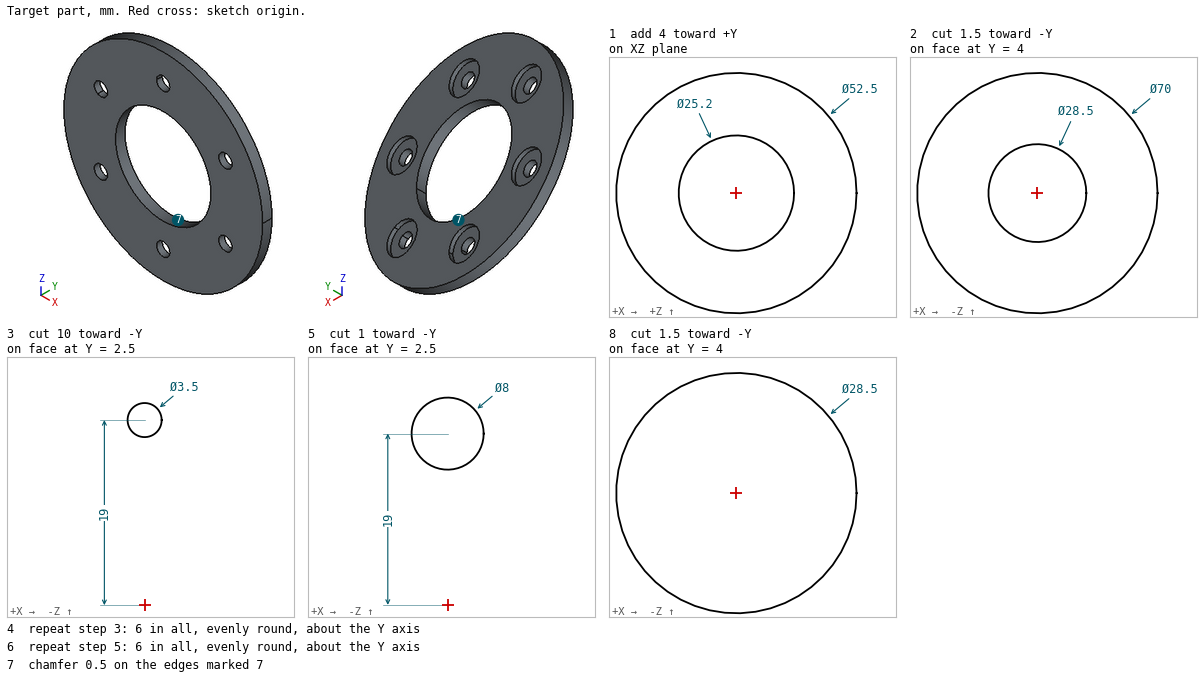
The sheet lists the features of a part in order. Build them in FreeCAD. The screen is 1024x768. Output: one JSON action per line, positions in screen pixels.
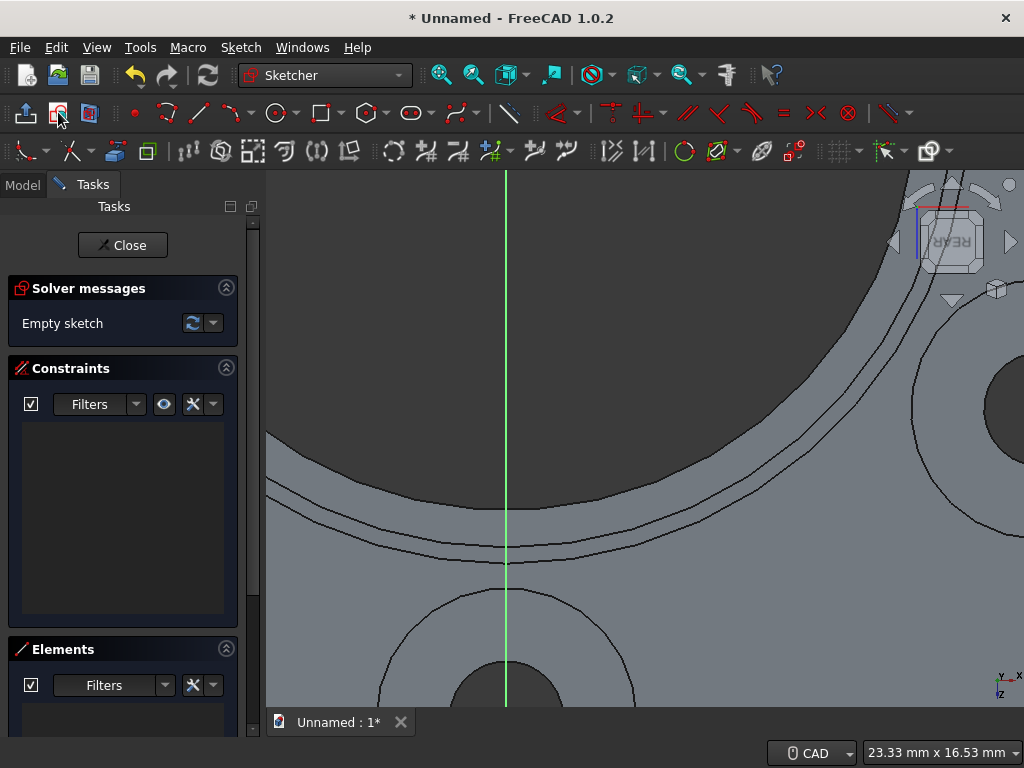
{"action": "scroll", "coordinate": [617, 635], "scroll_direction": "down", "scroll_amount": 5}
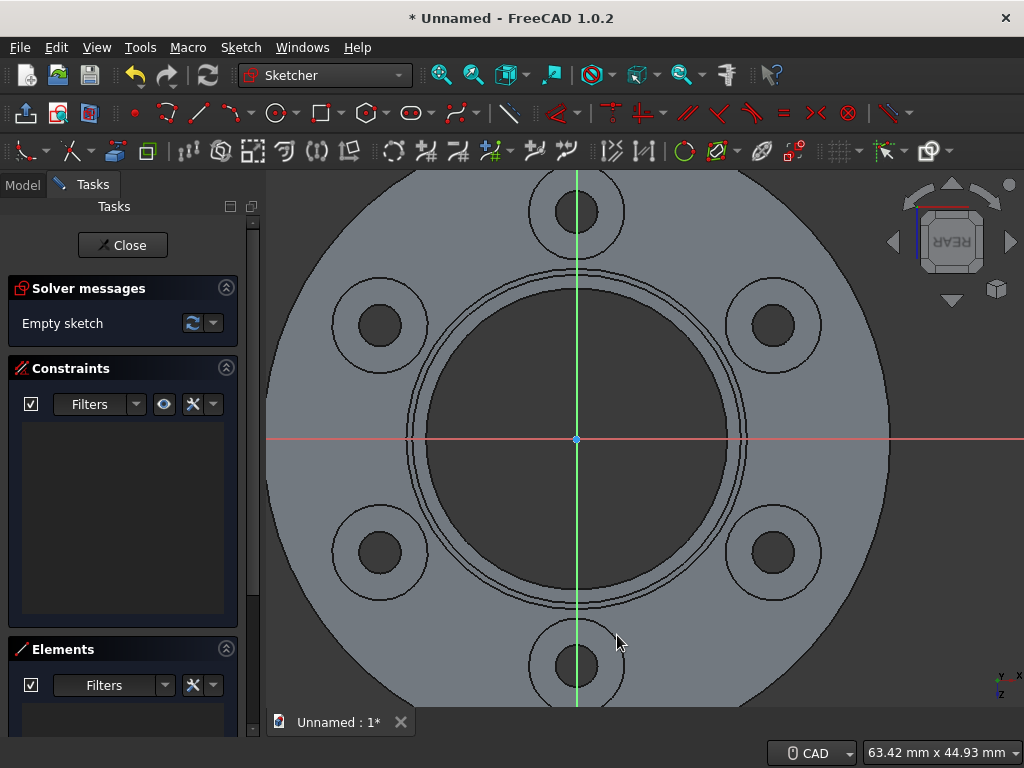
{"action": "left_click", "coordinate": [276, 114]}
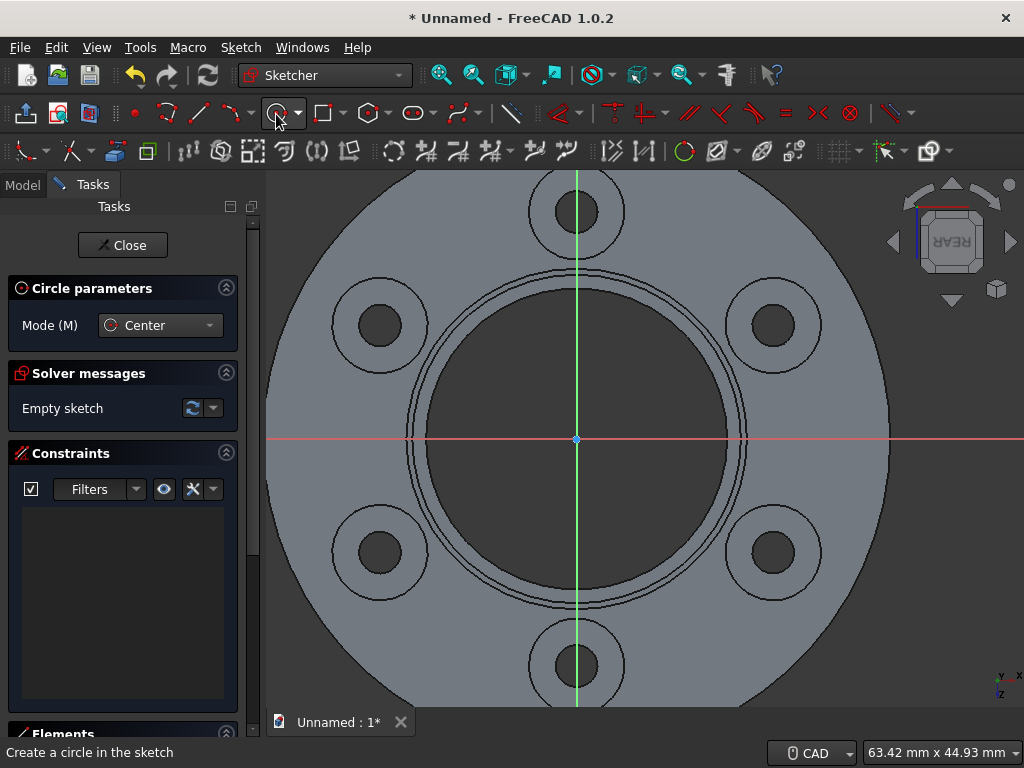
{"action": "left_click", "coordinate": [577, 439]}
{"action": "mouse_move", "coordinate": [697, 319]}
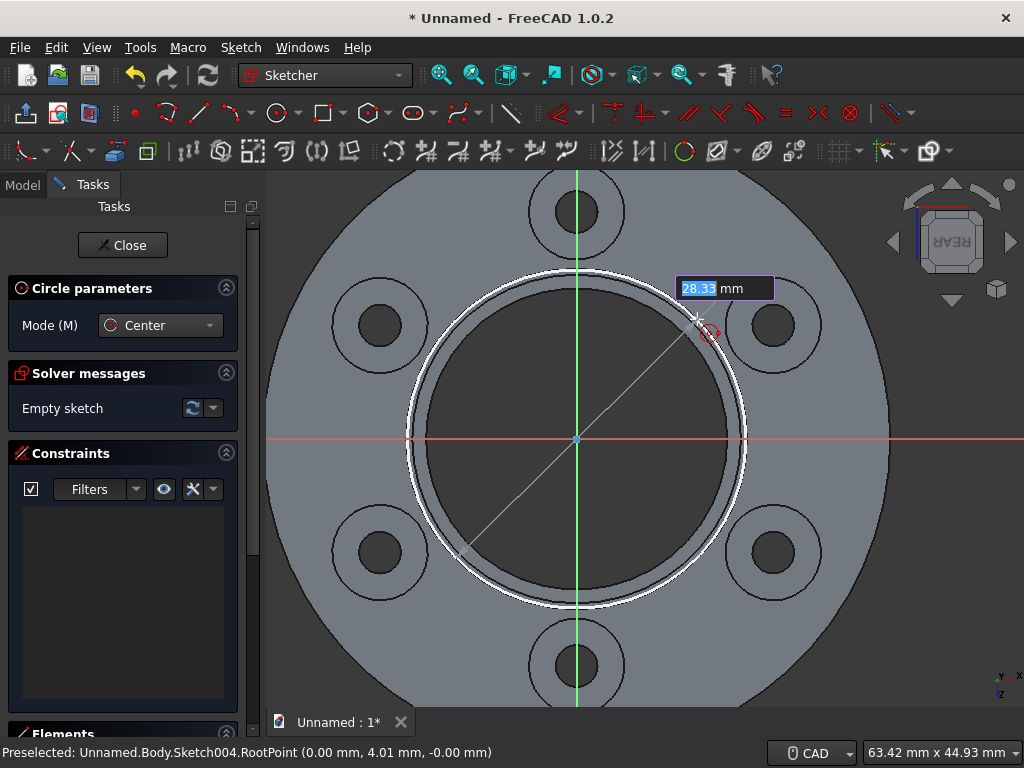
{"action": "type", "text": "28.5"}
{"action": "key", "text": "Return"}
{"action": "key", "text": "Escape"}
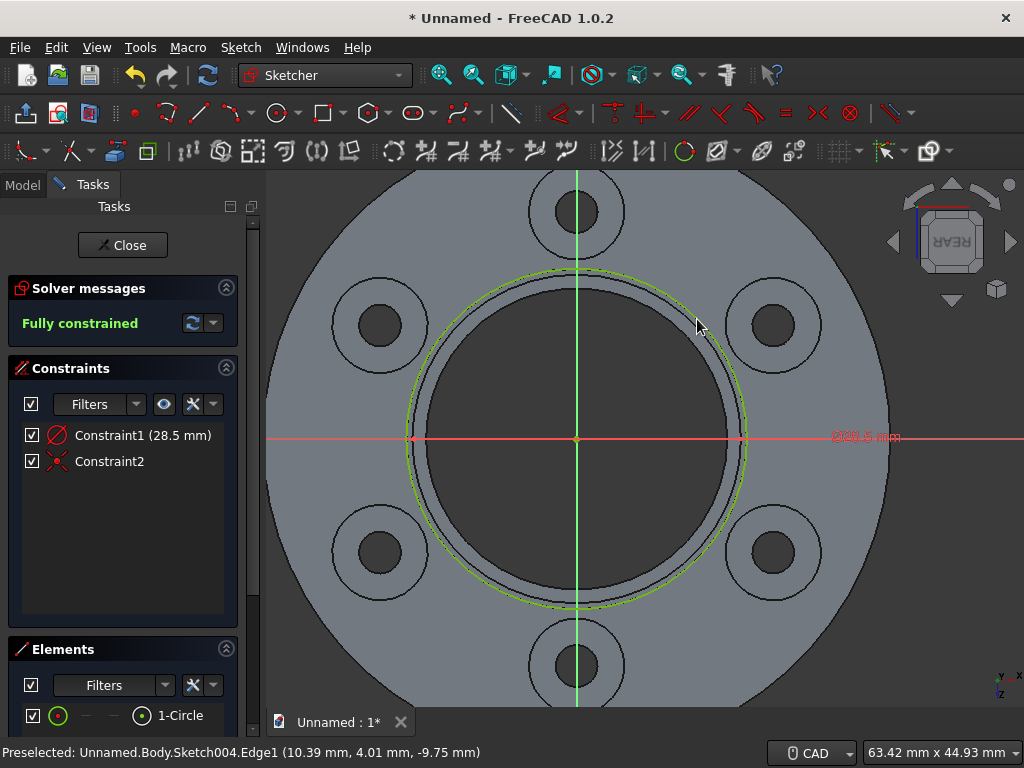
{"action": "left_click", "coordinate": [123, 245]}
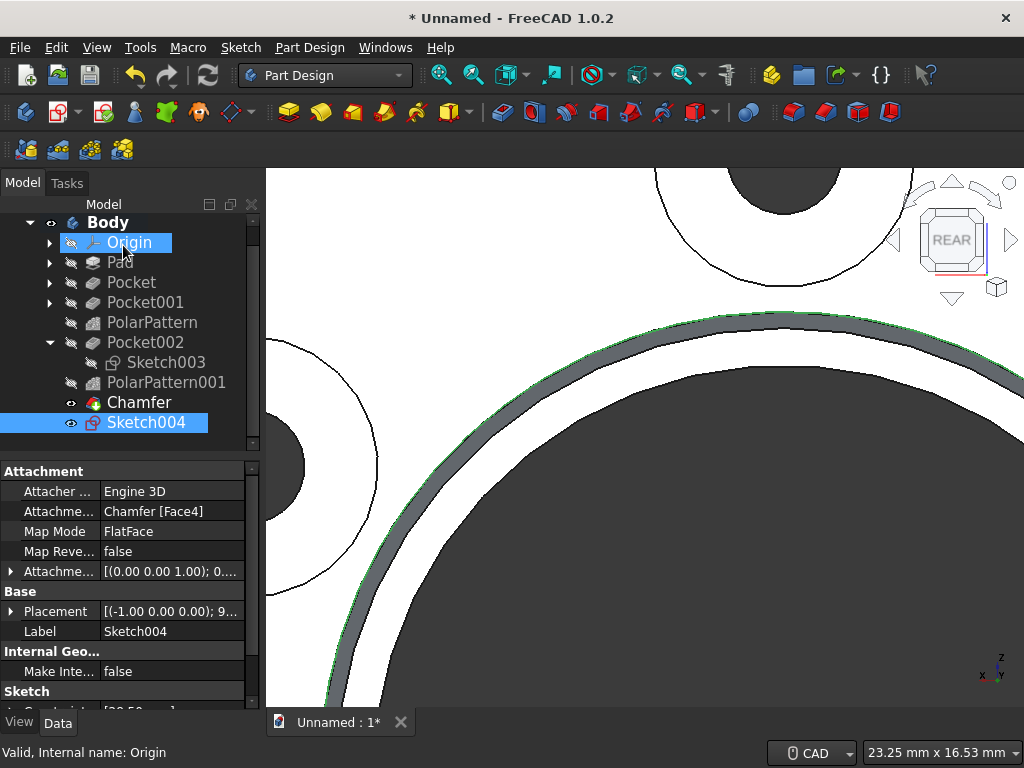
{"action": "left_click", "coordinate": [504, 112]}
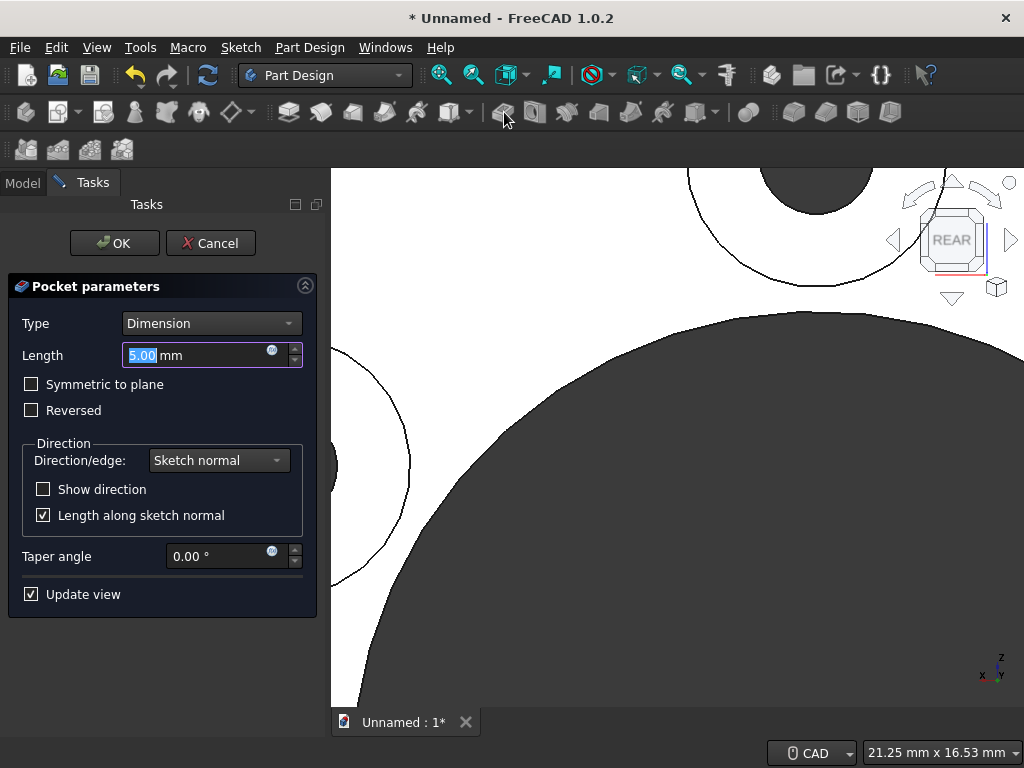
{"action": "type", "text": "1.5"}
{"action": "key", "text": "Tab"}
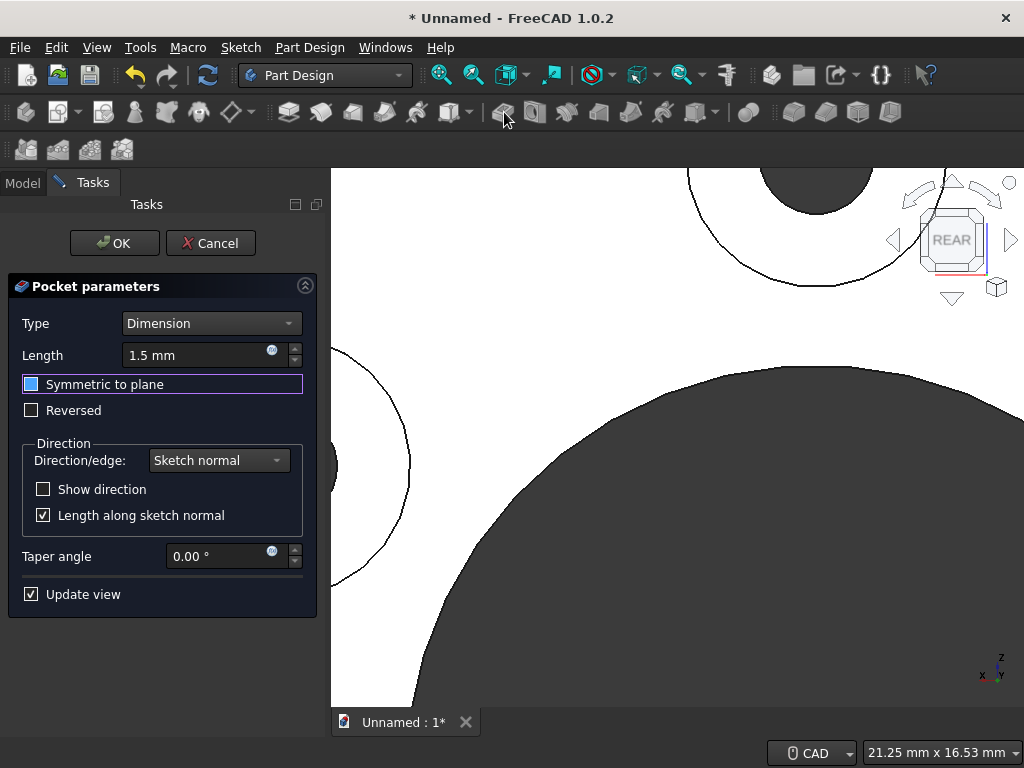
{"action": "left_click", "coordinate": [115, 243]}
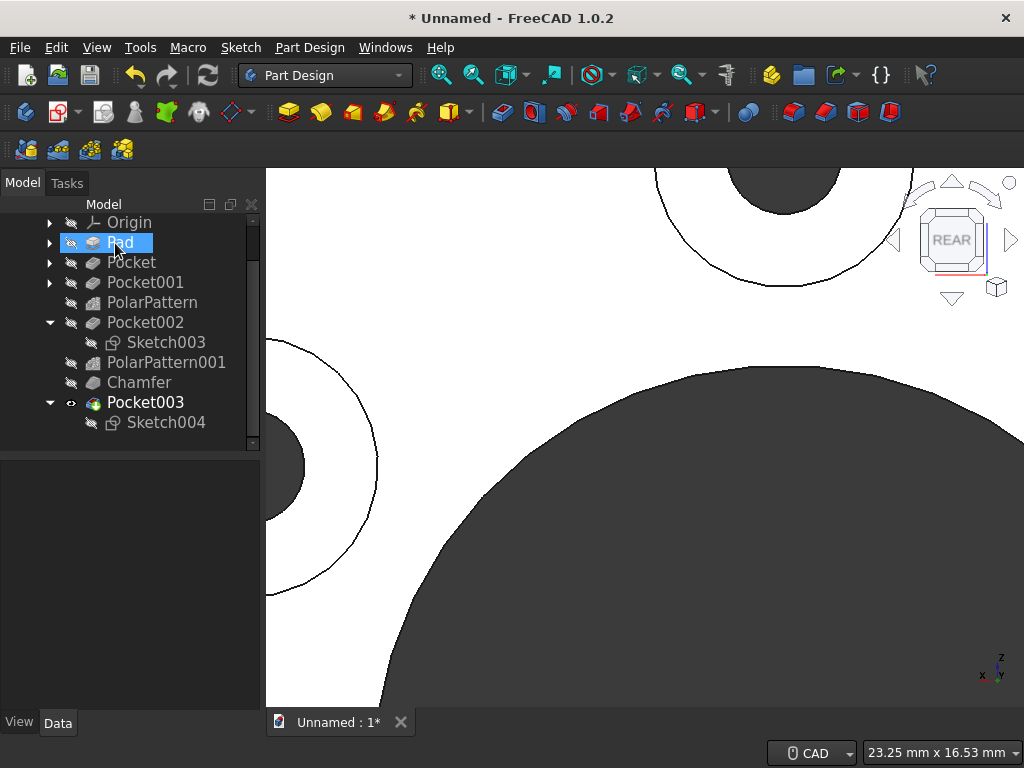
{"action": "key", "text": "0"}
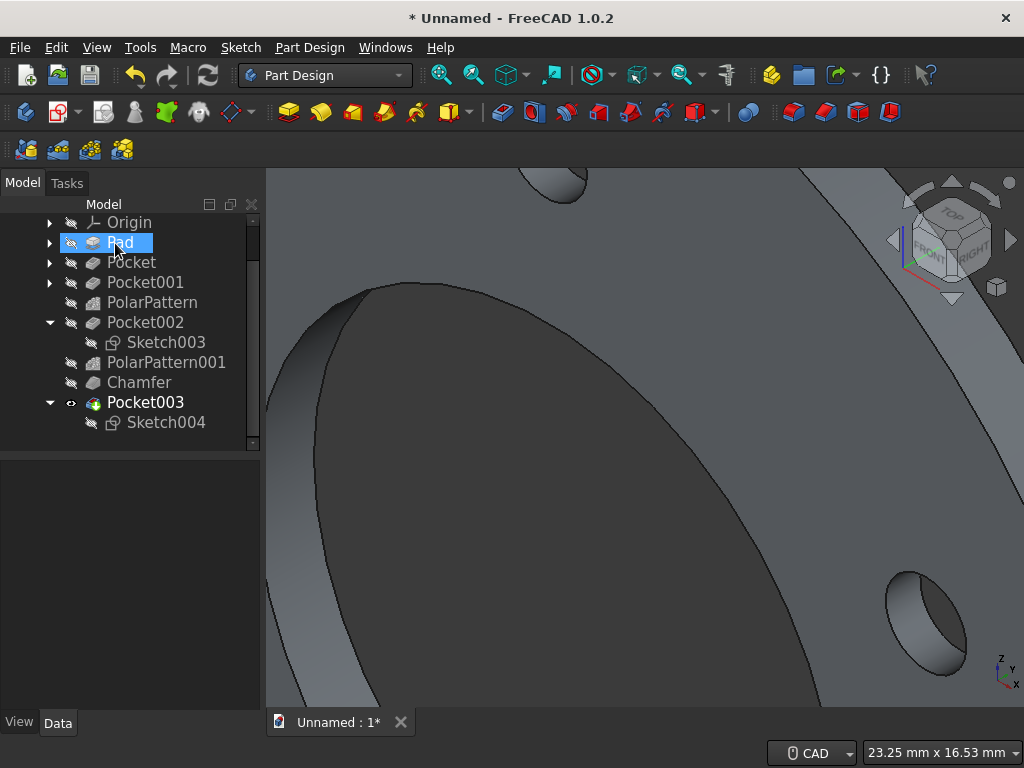
{"action": "left_click", "coordinate": [442, 76]}